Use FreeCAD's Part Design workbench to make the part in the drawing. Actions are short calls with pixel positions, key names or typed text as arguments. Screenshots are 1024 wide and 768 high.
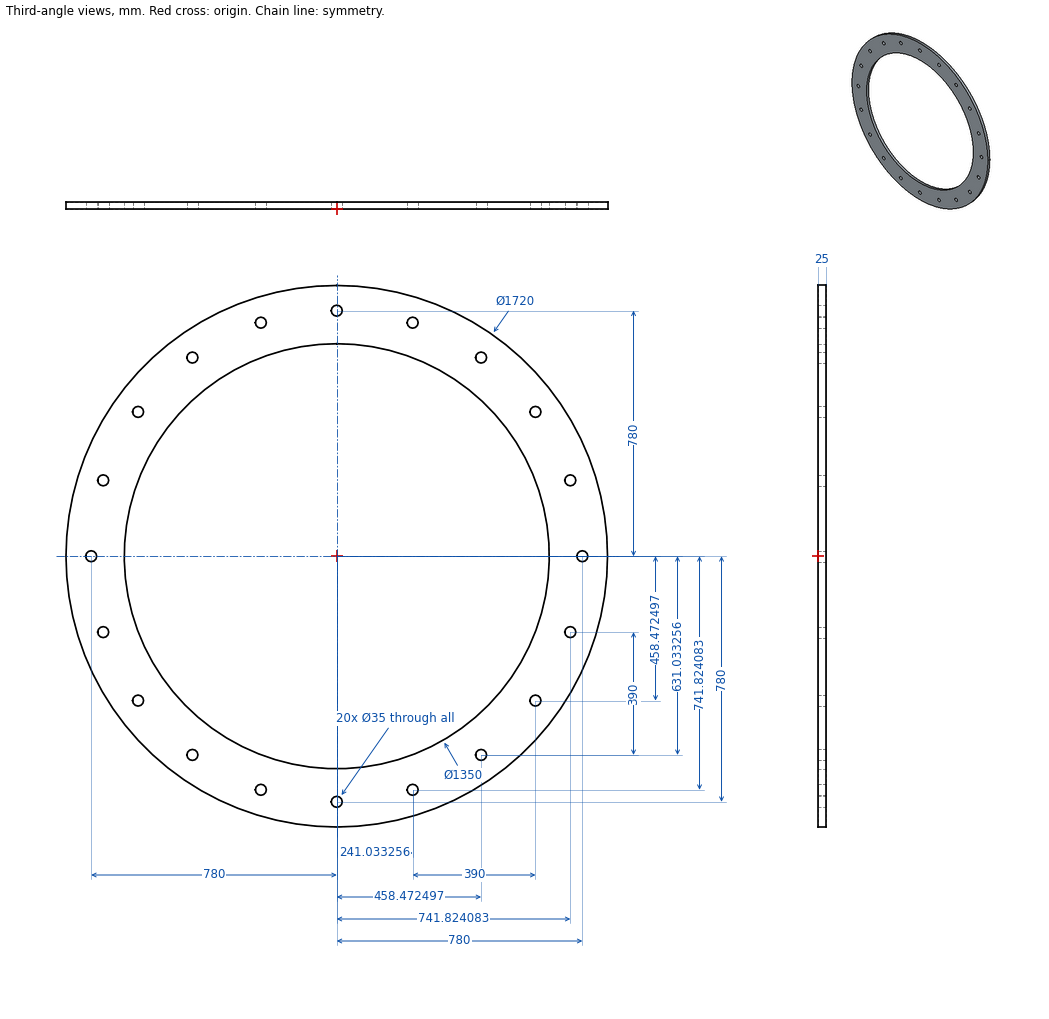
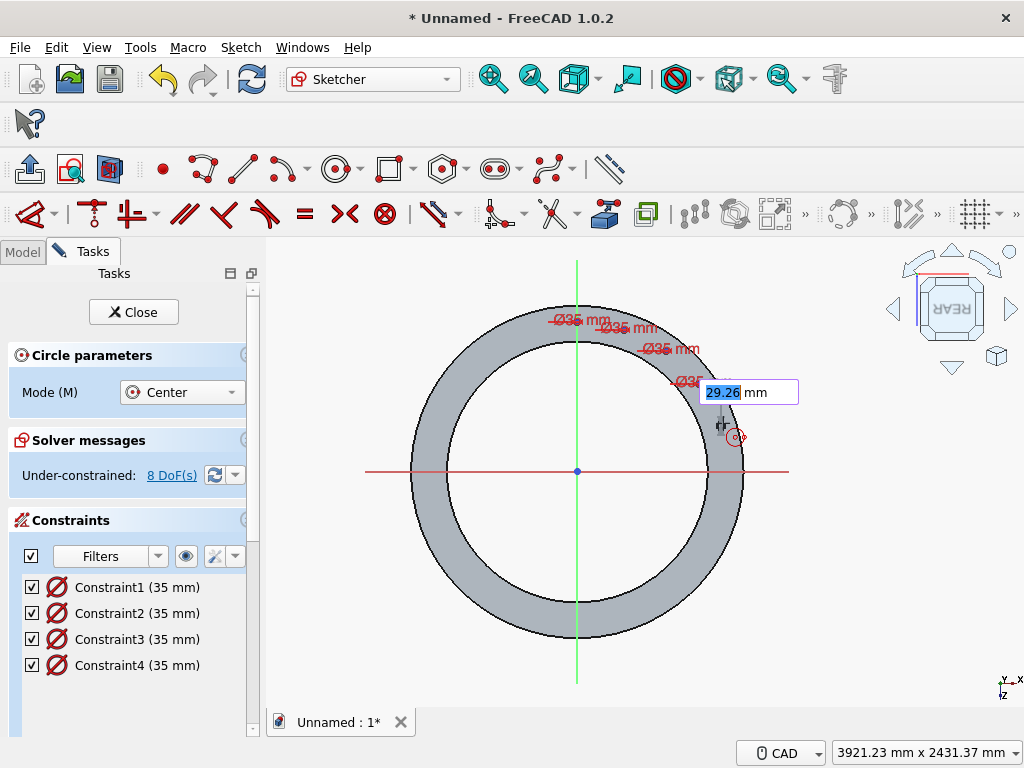
text(35)
key(Return)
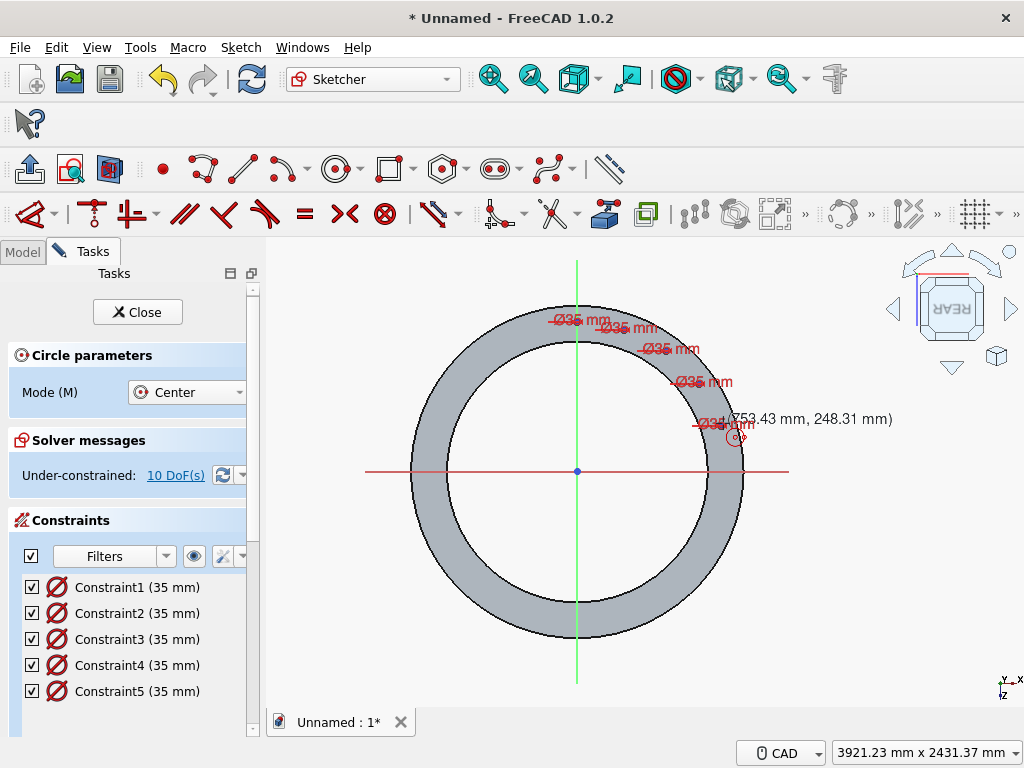
scroll(728, 472, up, 10)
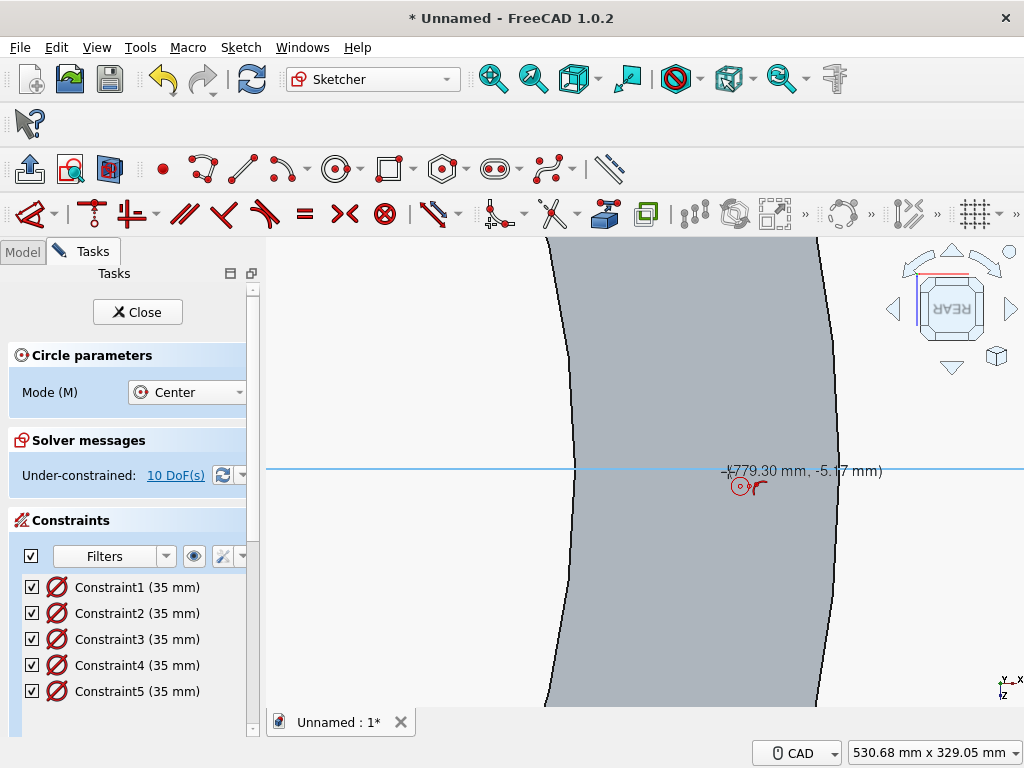
scroll(728, 473, down, 10)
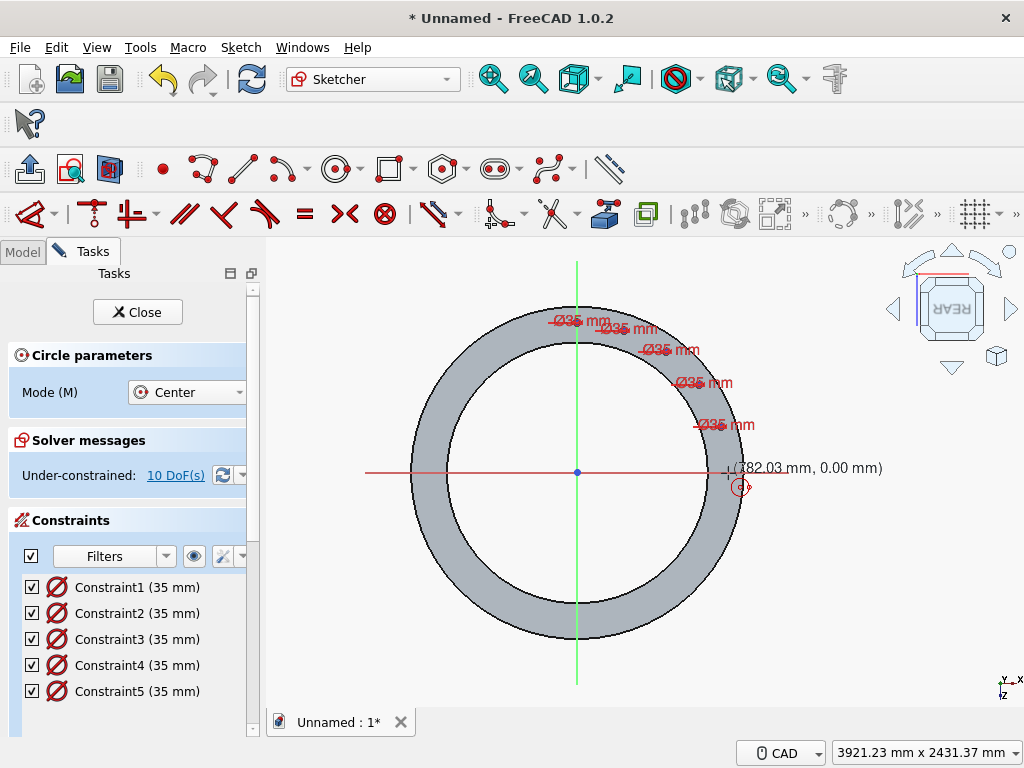
click(728, 473)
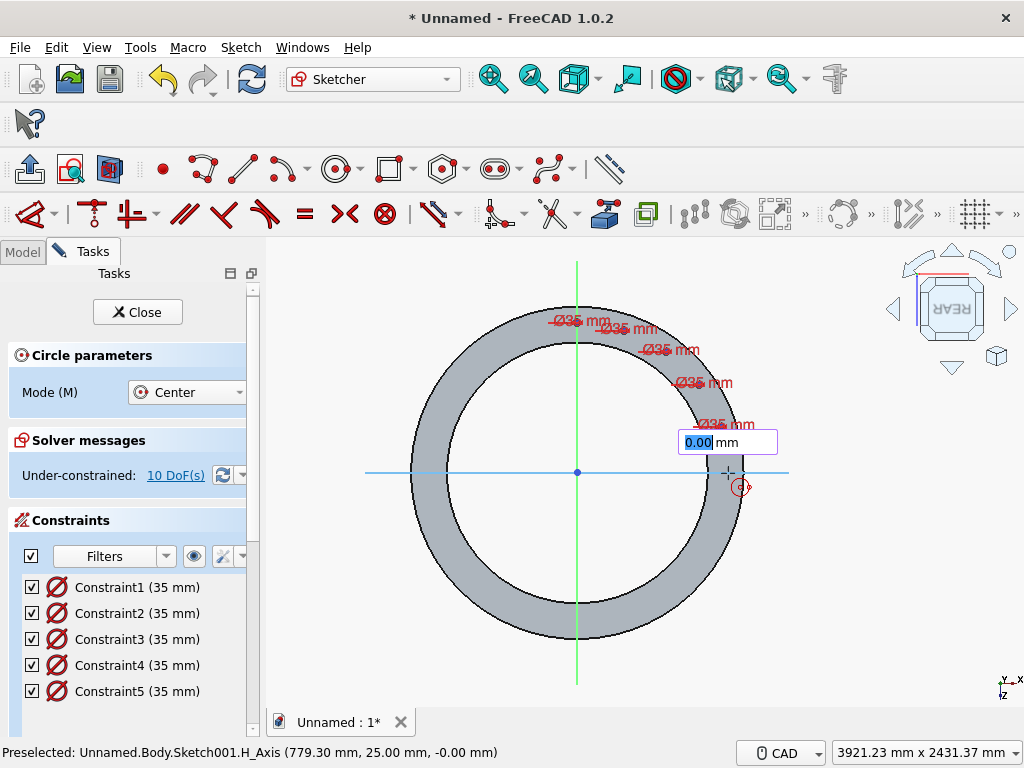
scroll(729, 470, up, 9)
move(728, 466)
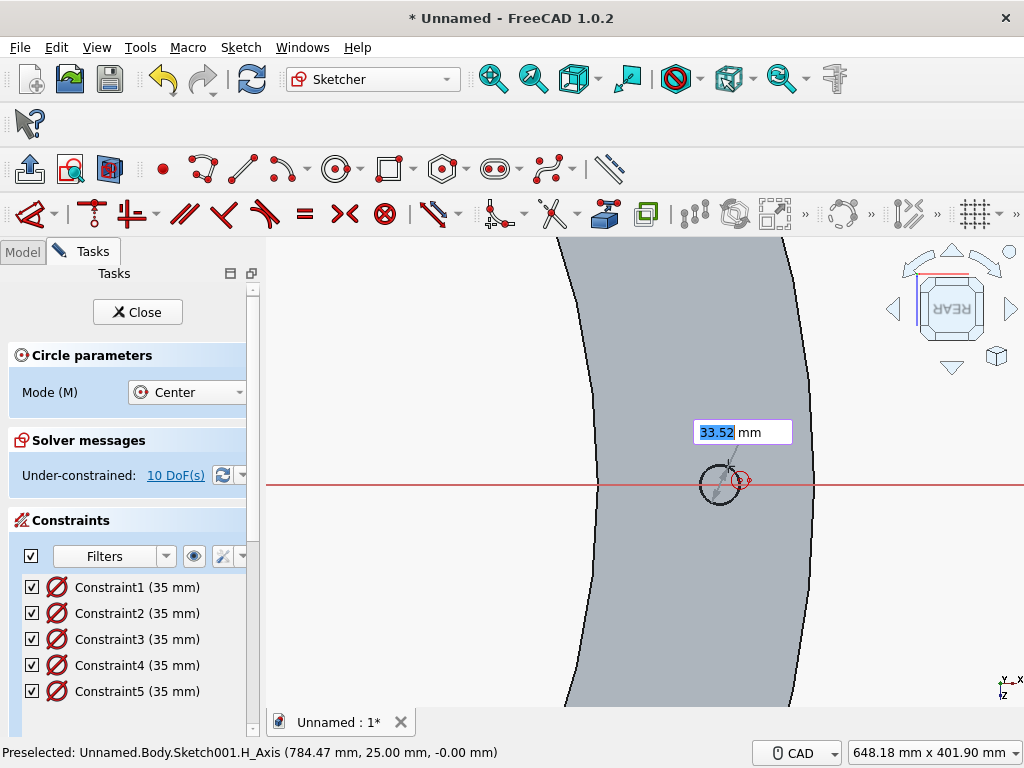
text(35)
key(Return)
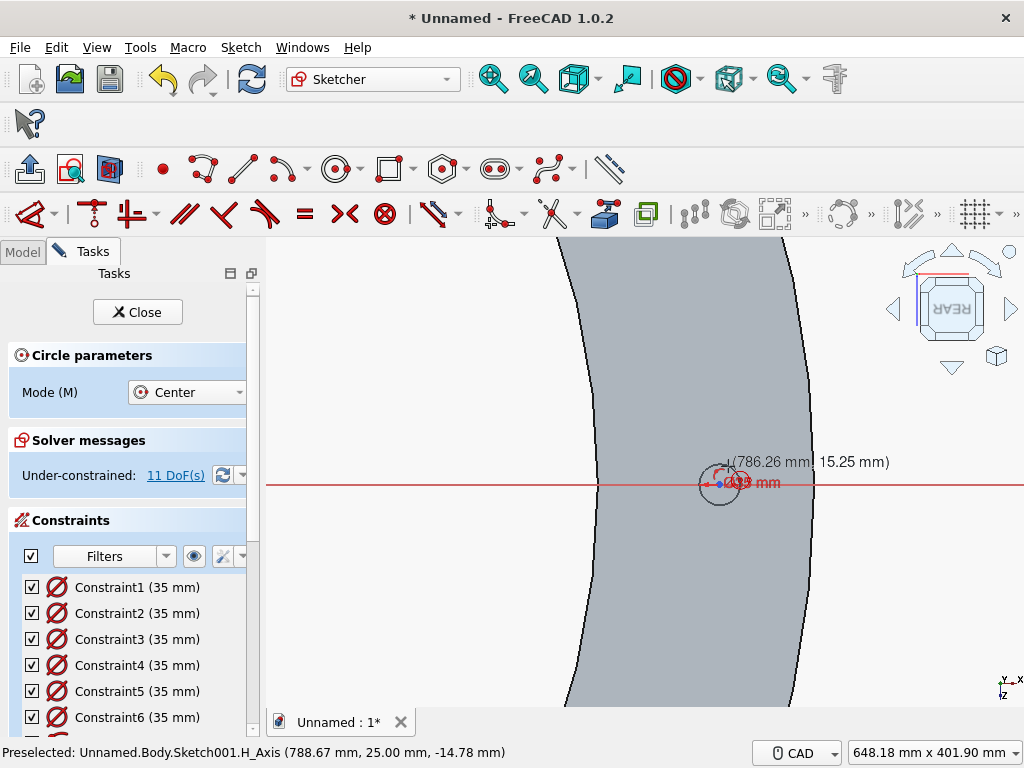
scroll(729, 469, down, 9)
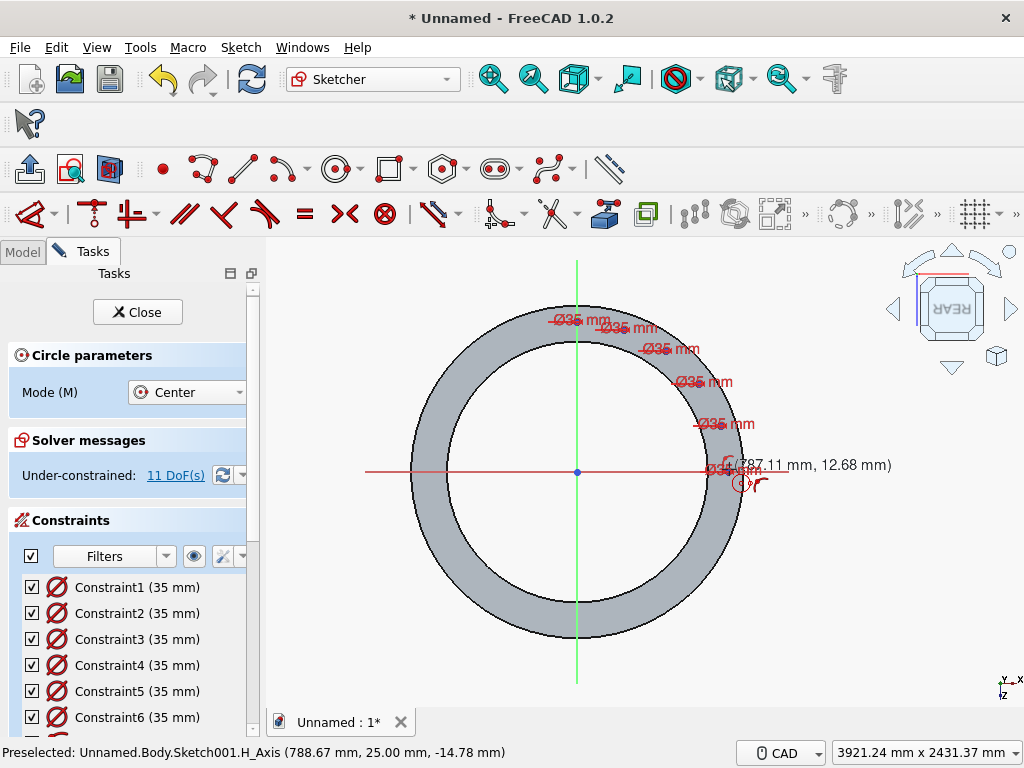
scroll(721, 519, up, 10)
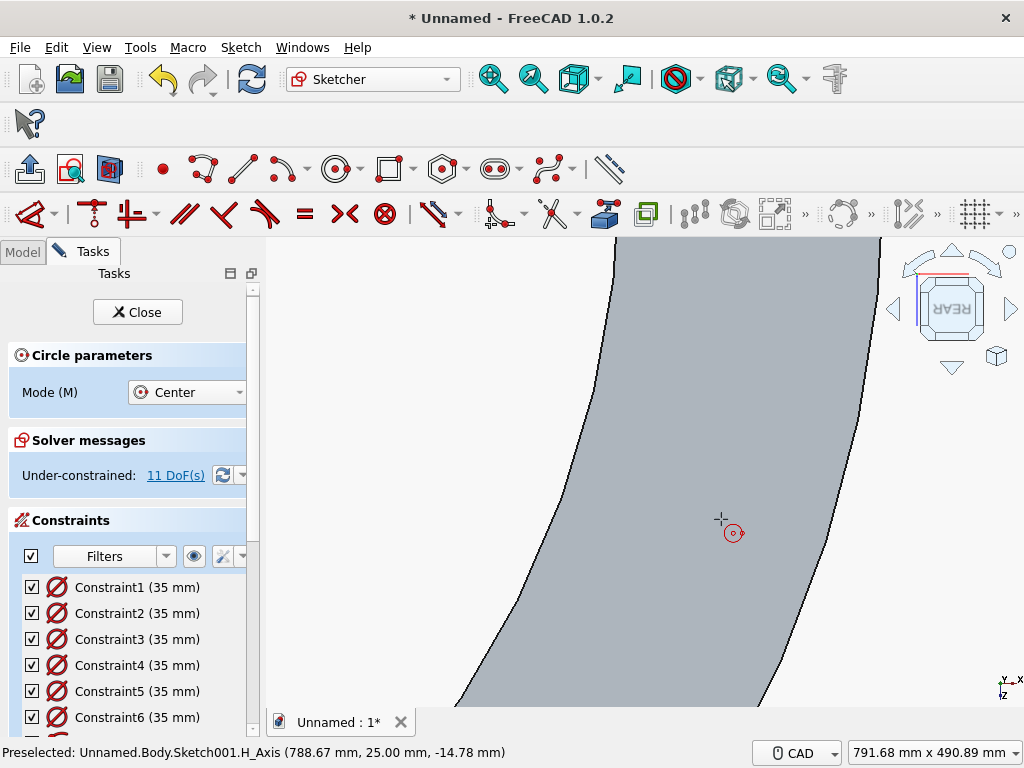
scroll(721, 520, down, 10)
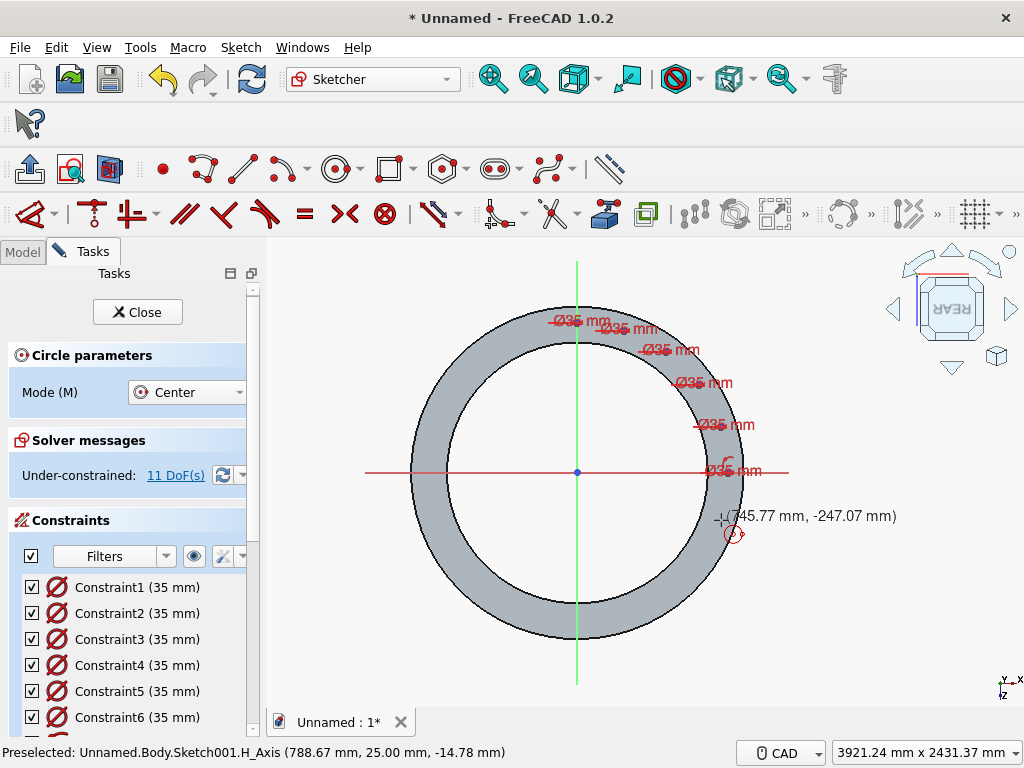
click(721, 519)
move(723, 517)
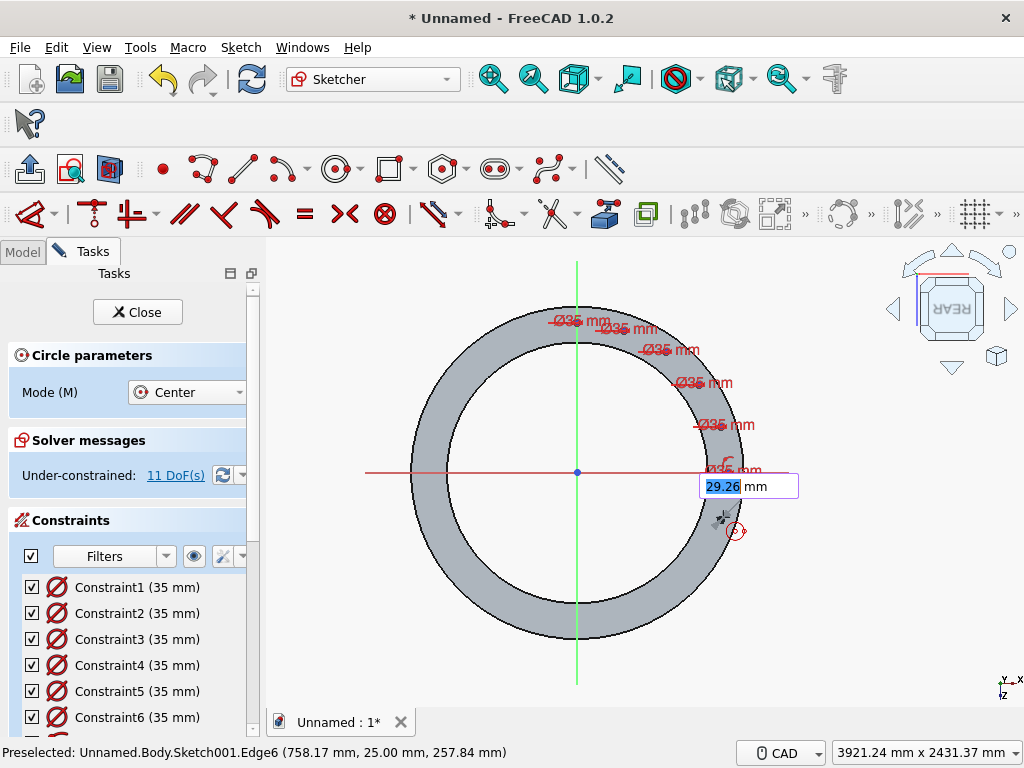
text(35)
key(Return)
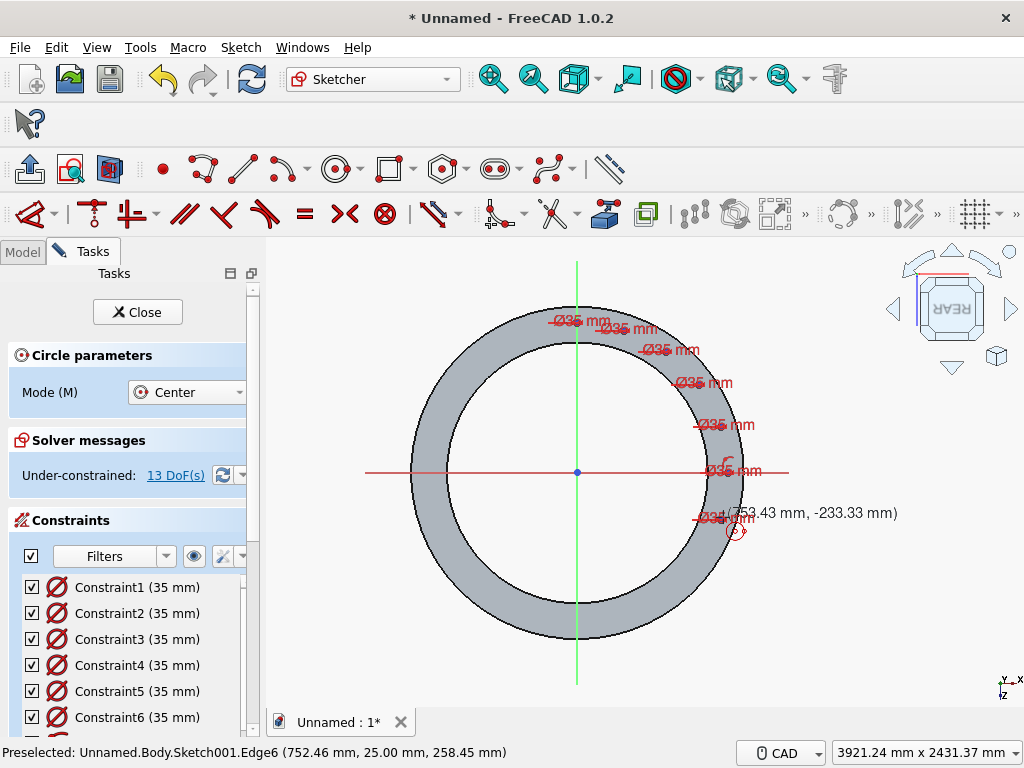
scroll(699, 562, up, 10)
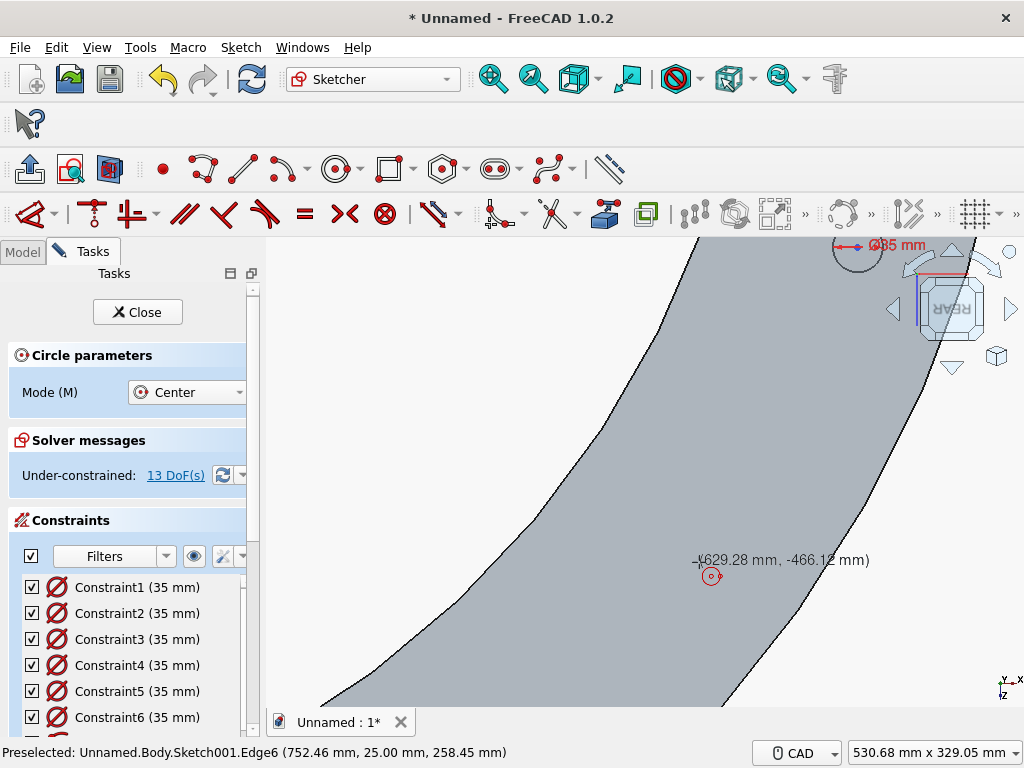
scroll(699, 562, down, 10)